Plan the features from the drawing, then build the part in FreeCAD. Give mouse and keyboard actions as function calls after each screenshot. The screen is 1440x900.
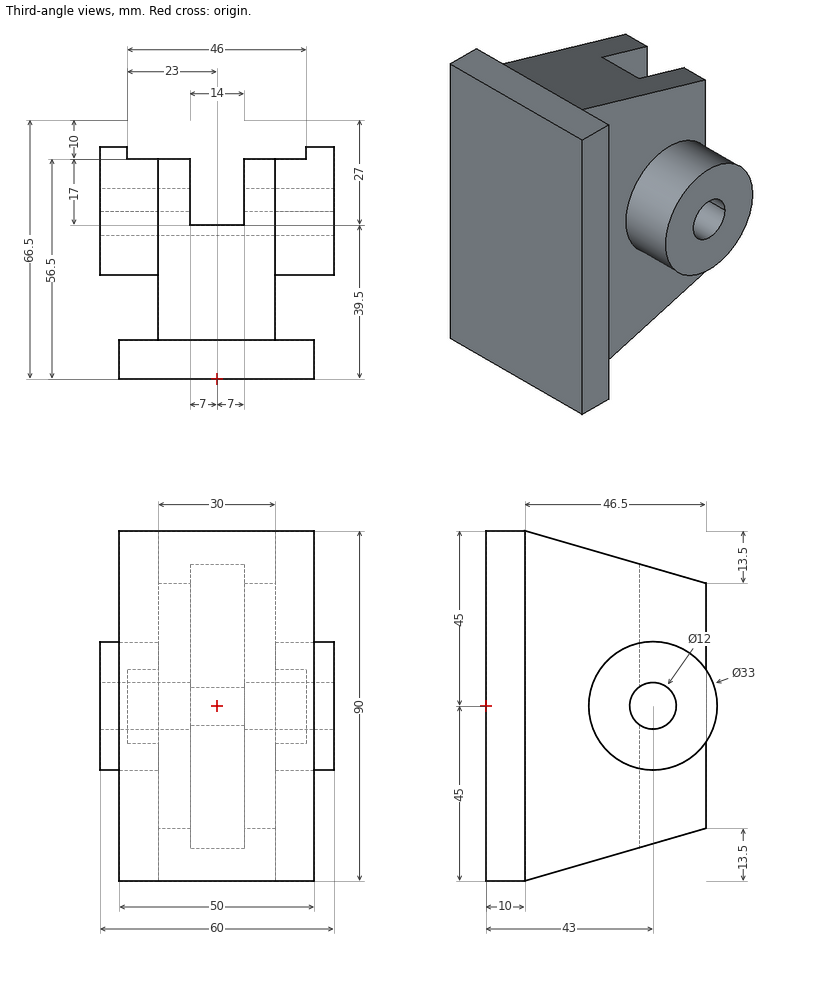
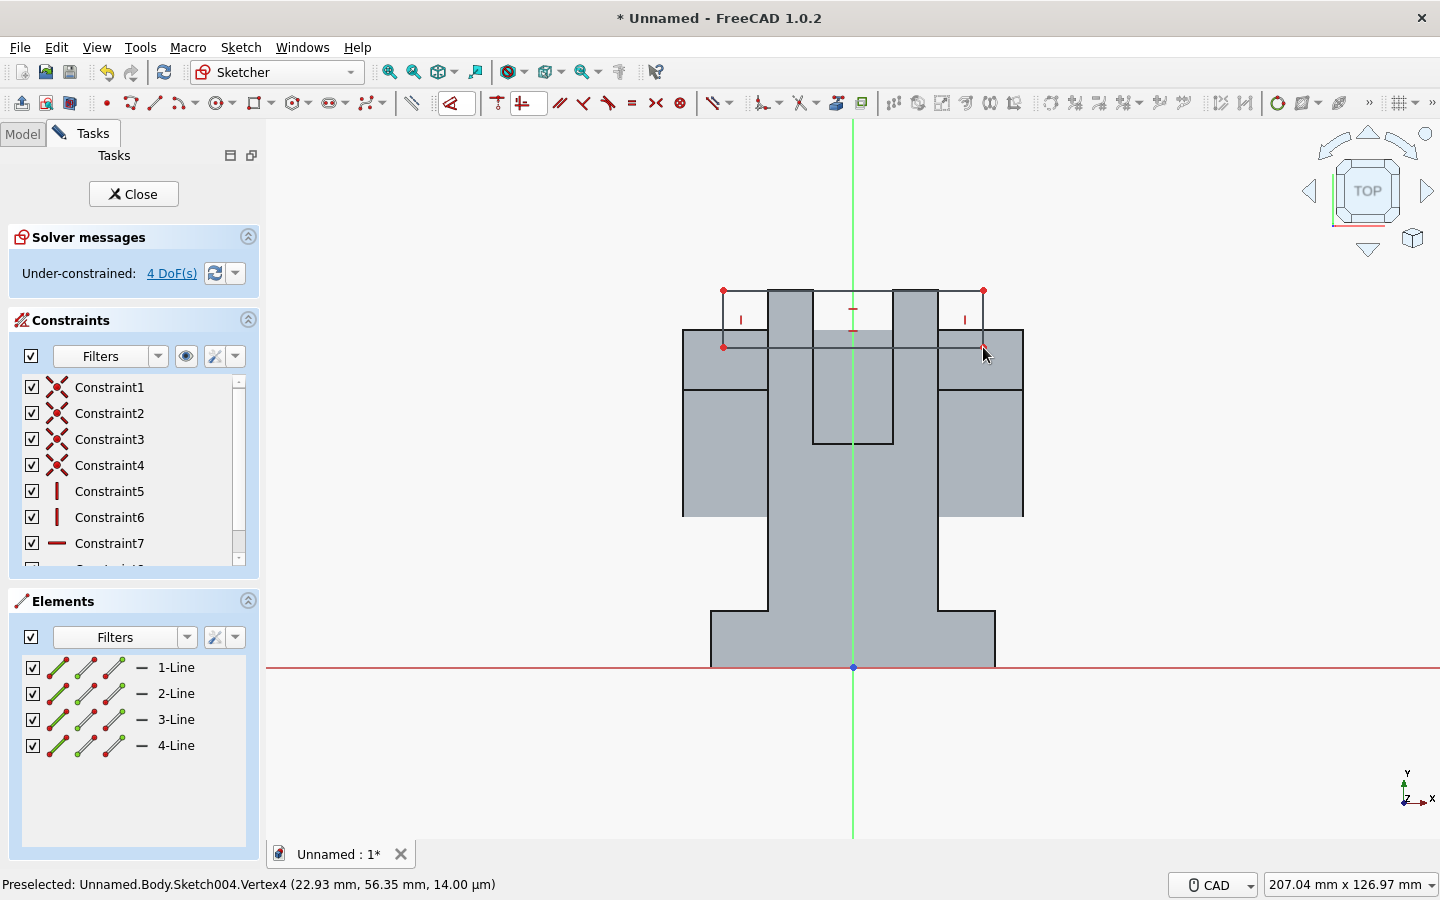
click(723, 308)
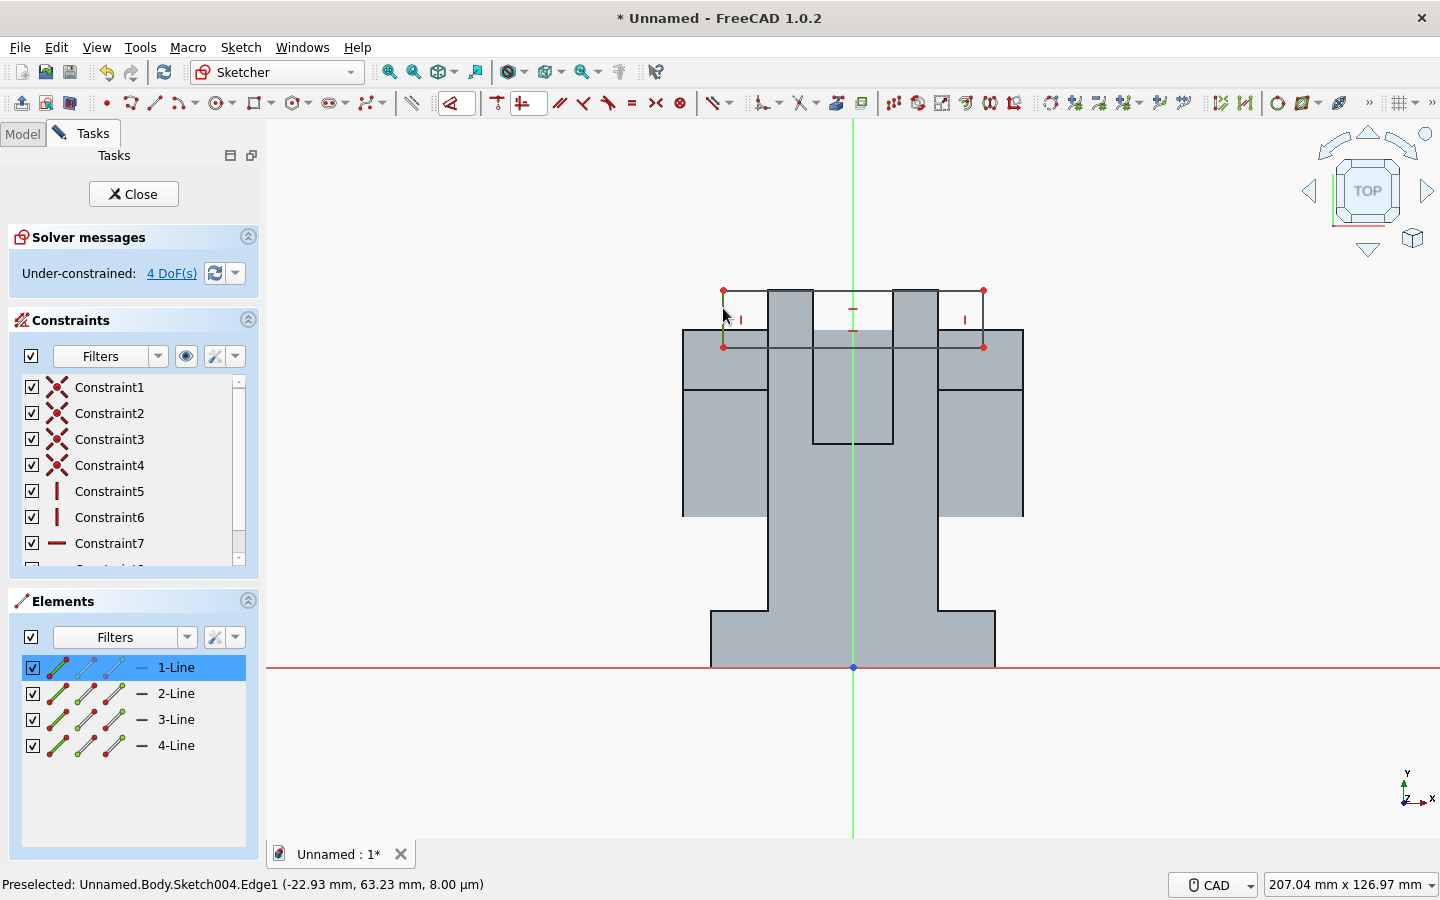
click(470, 104)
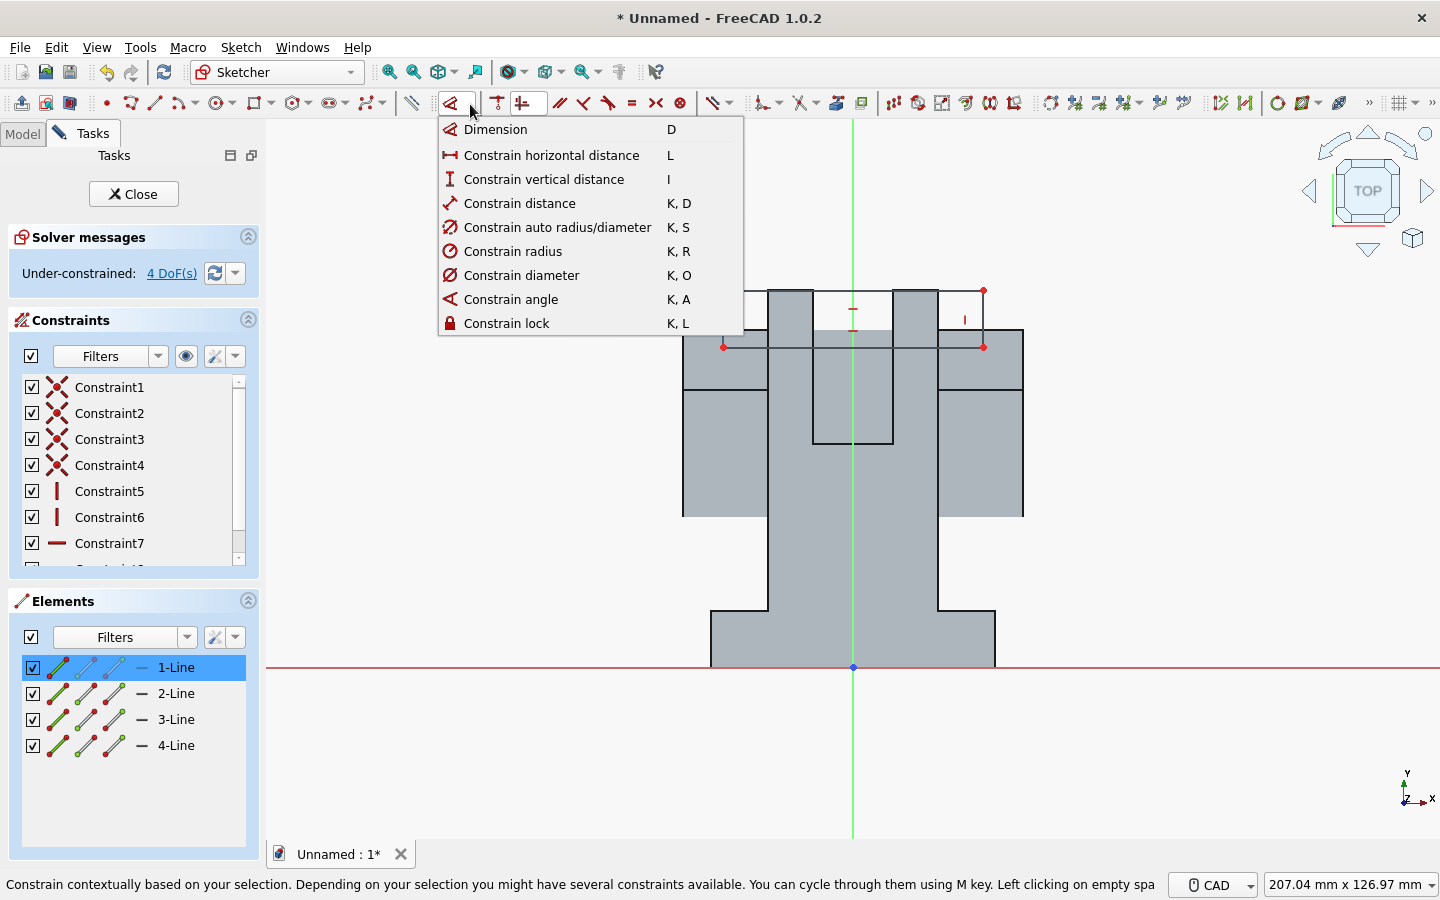
click(591, 179)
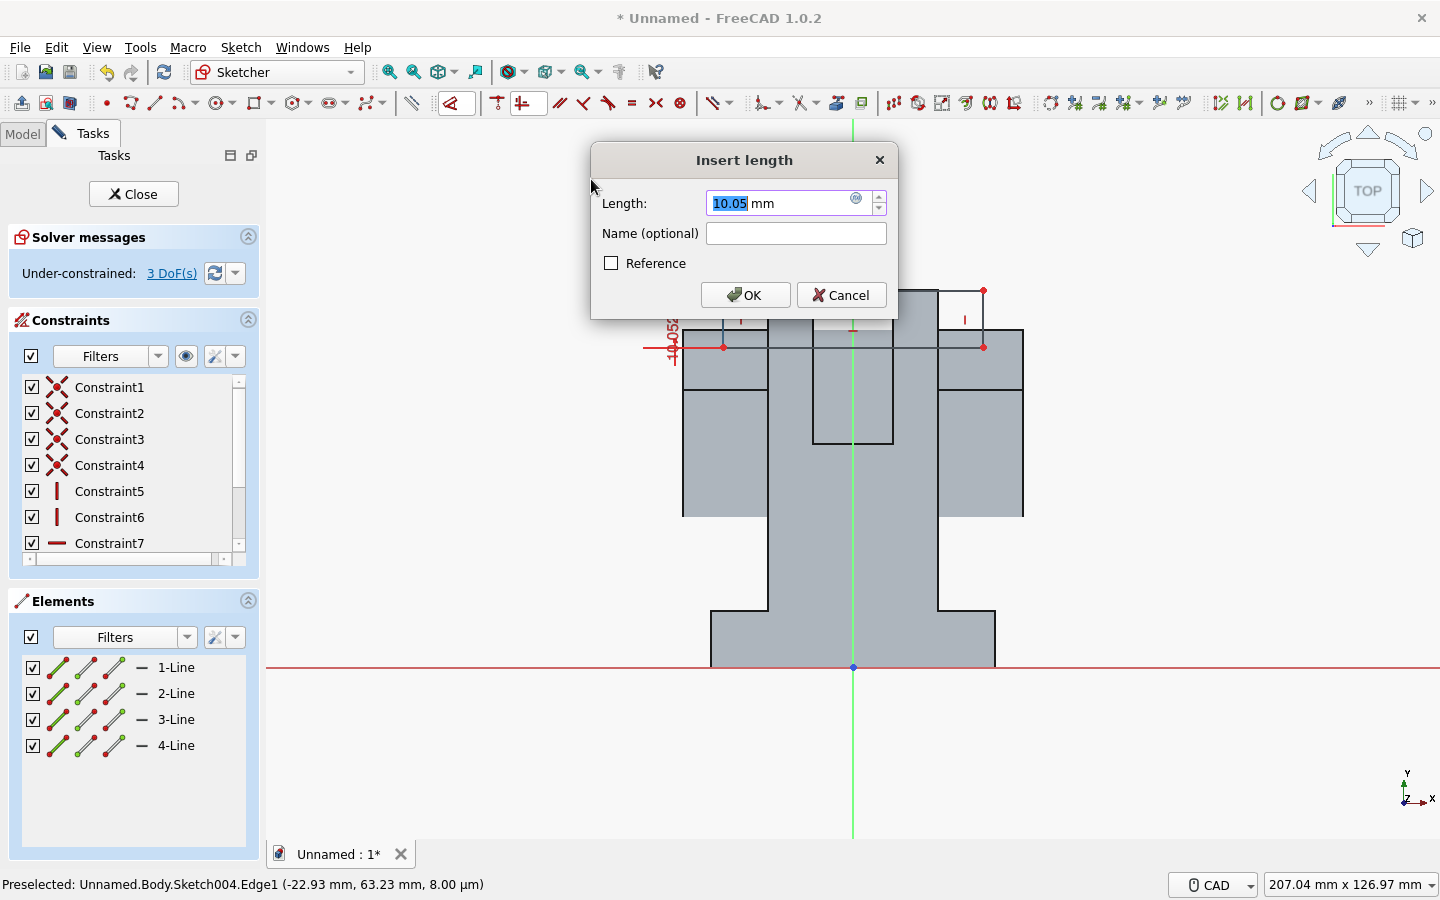
text(10)
key(Return)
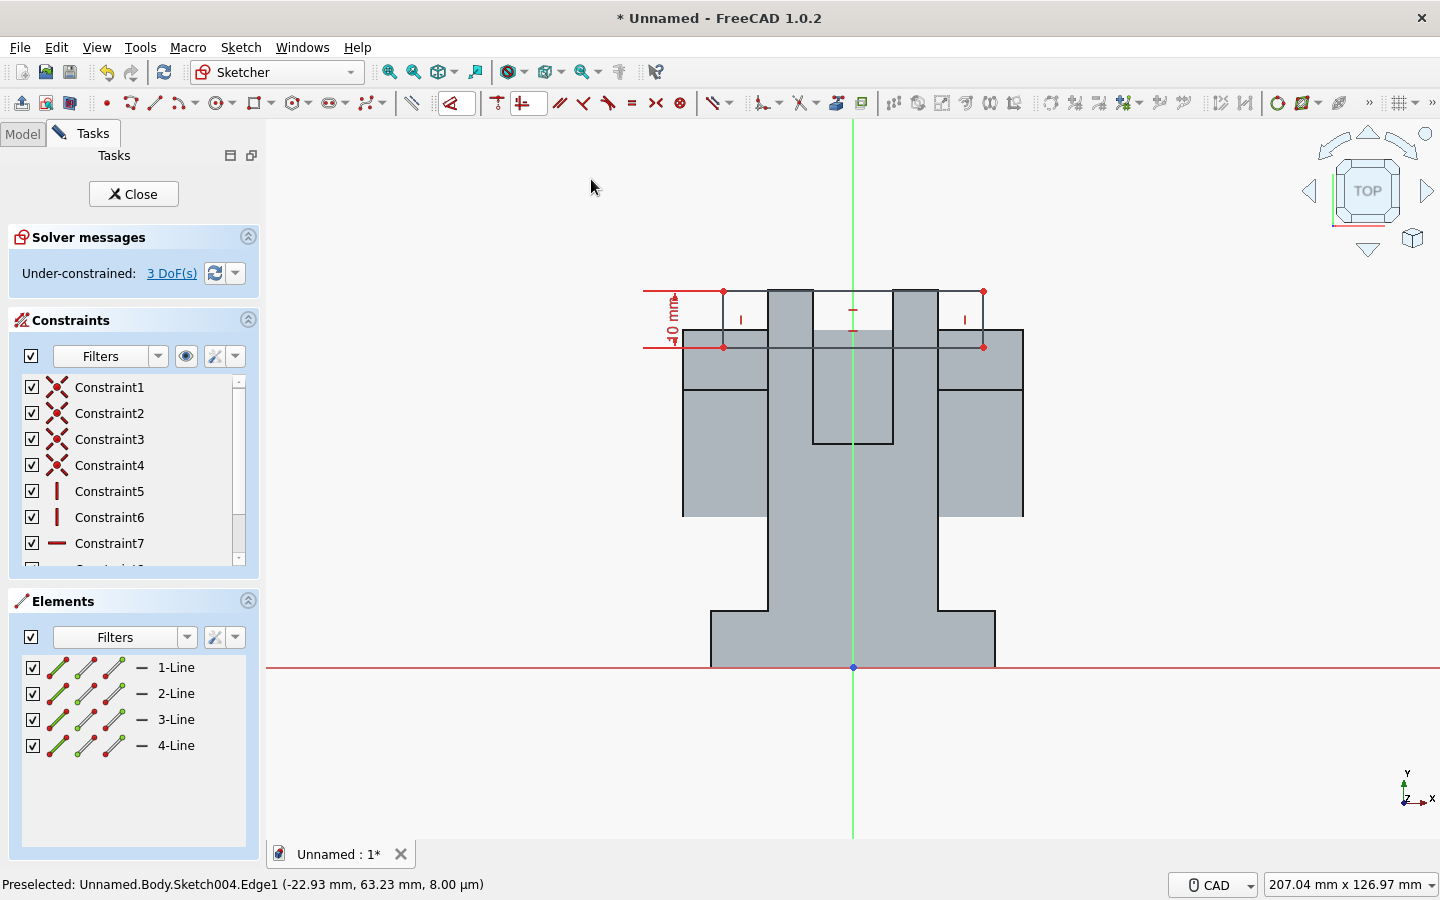
click(801, 348)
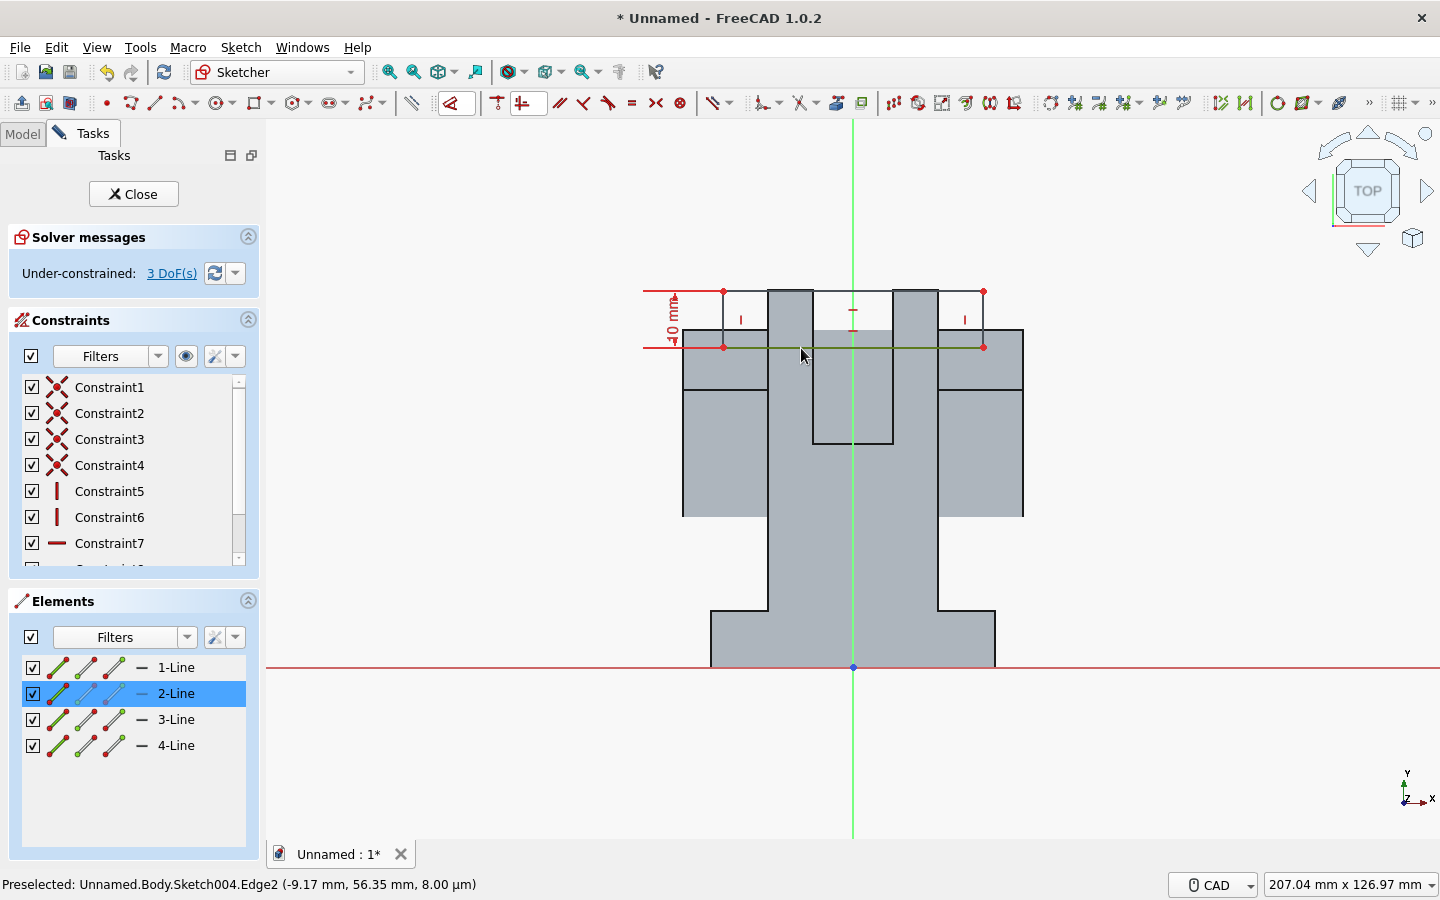
click(470, 104)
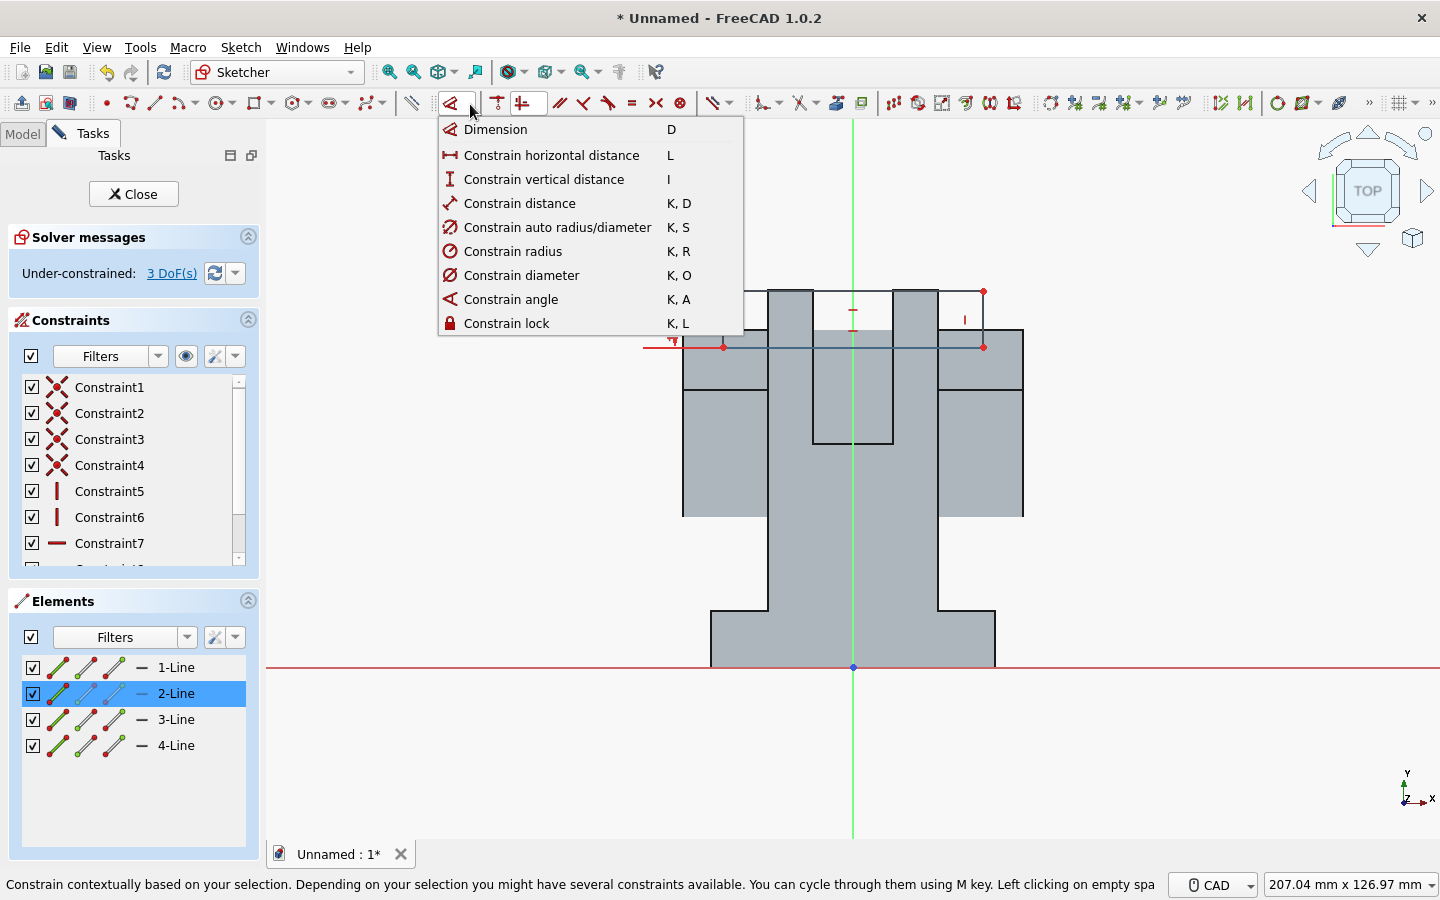
click(591, 155)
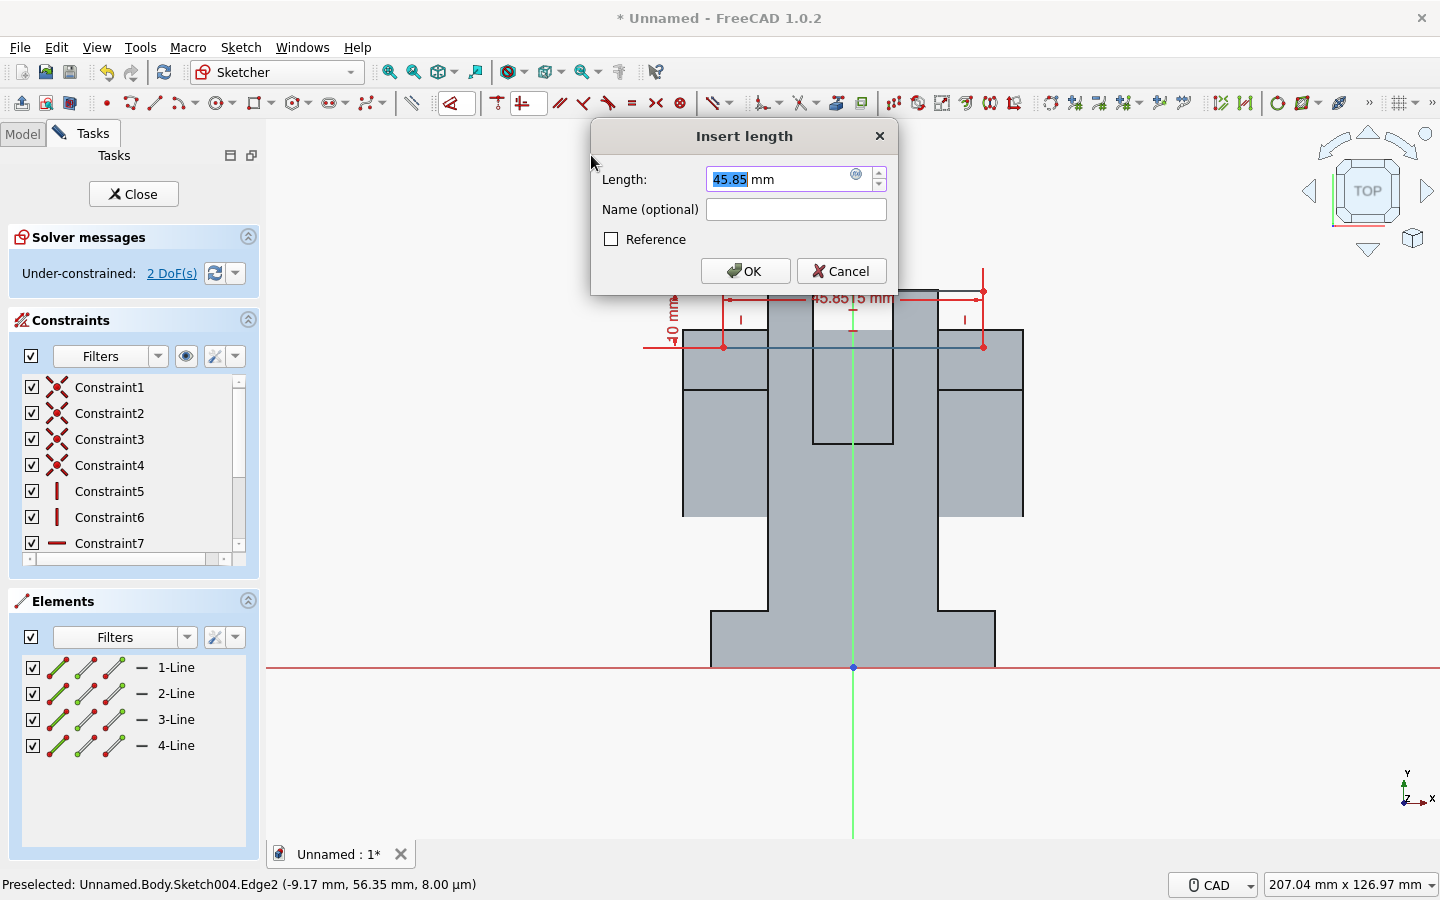
text(46)
key(Return)